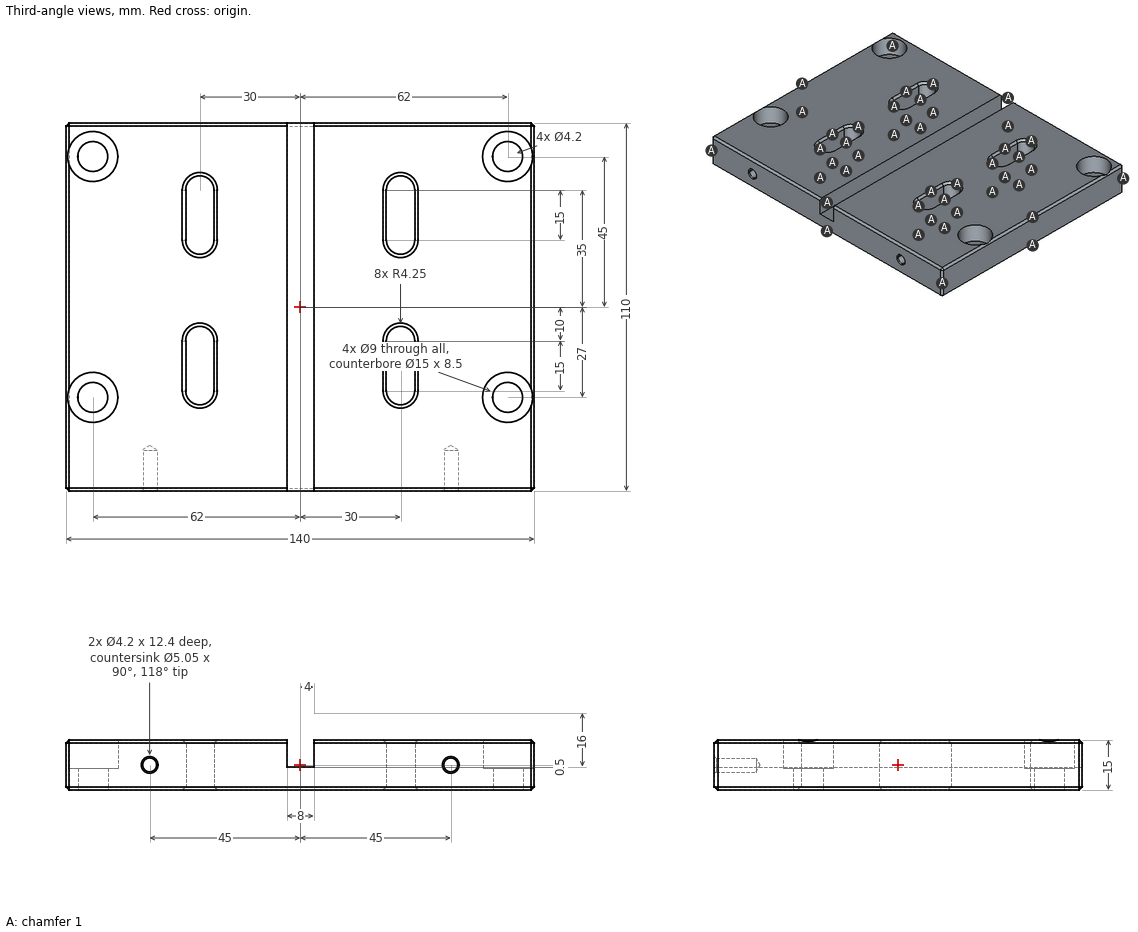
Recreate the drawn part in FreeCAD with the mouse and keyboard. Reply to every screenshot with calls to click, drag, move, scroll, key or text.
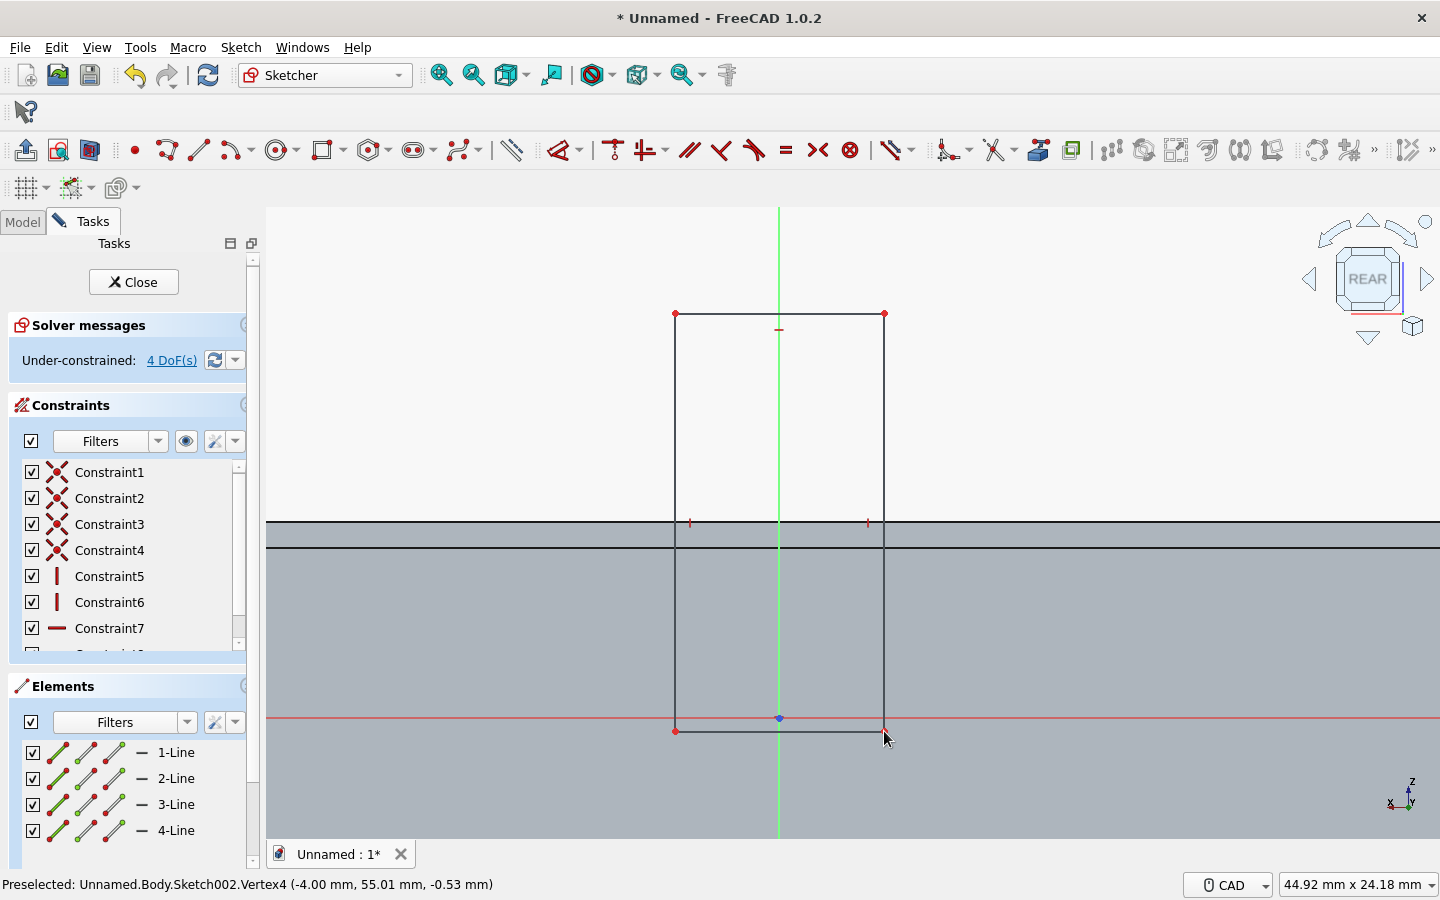
click(558, 150)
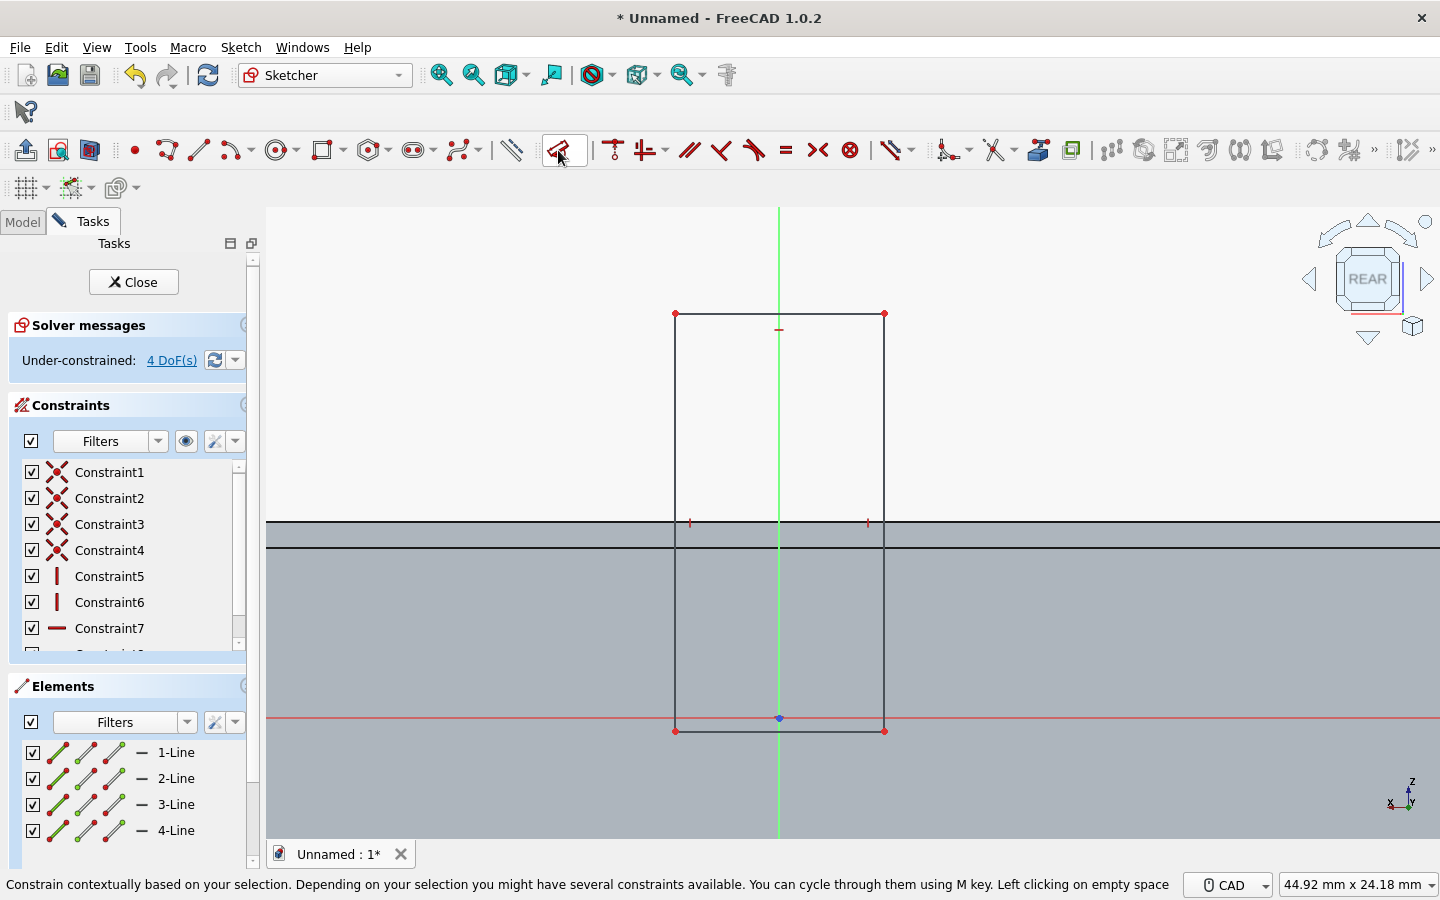
click(738, 732)
click(731, 766)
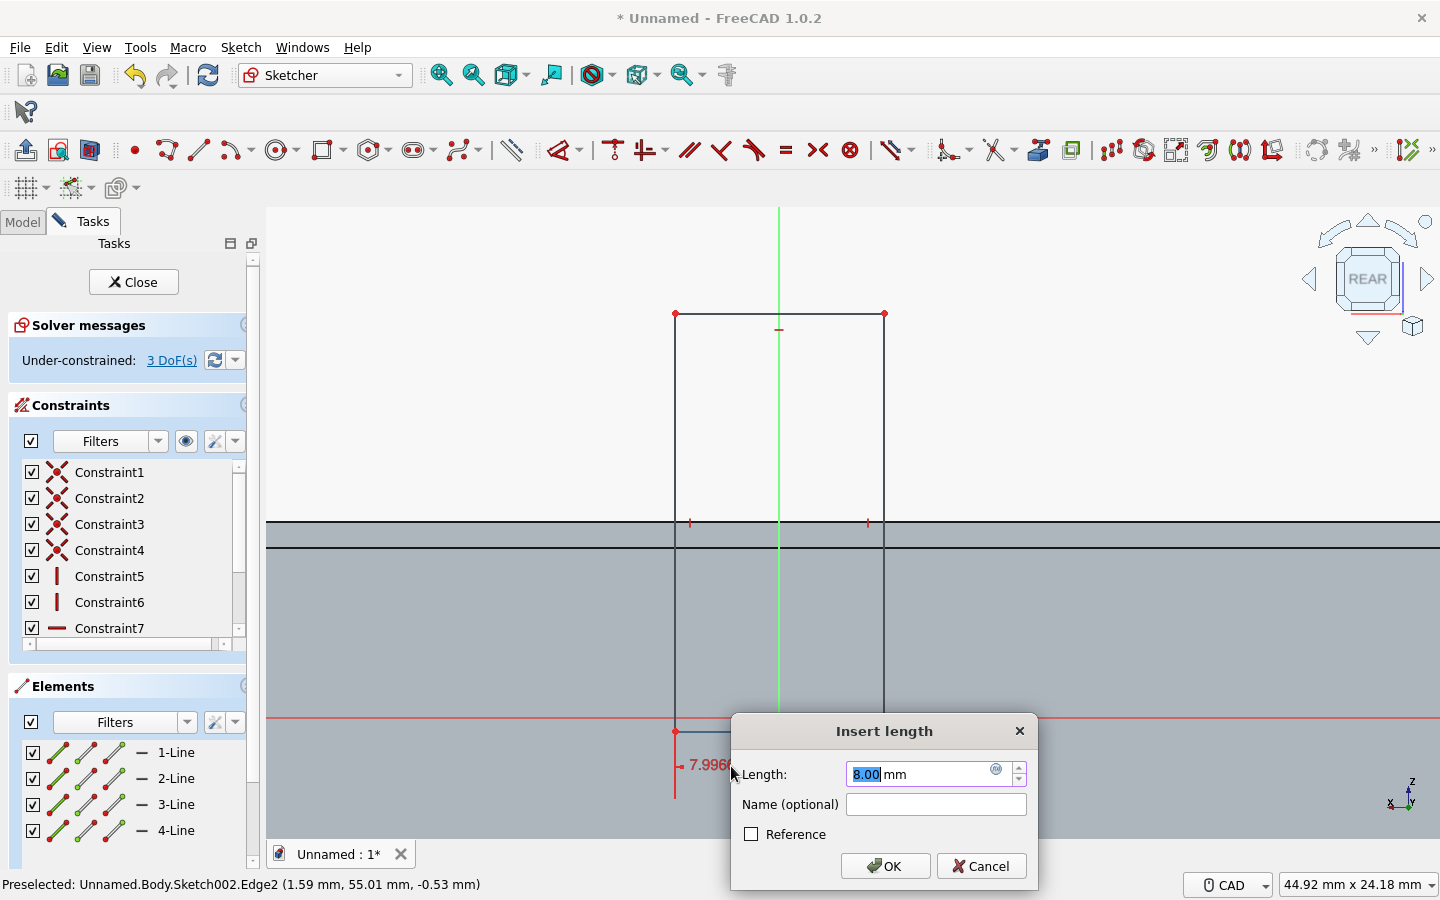
text(8)
key(Return)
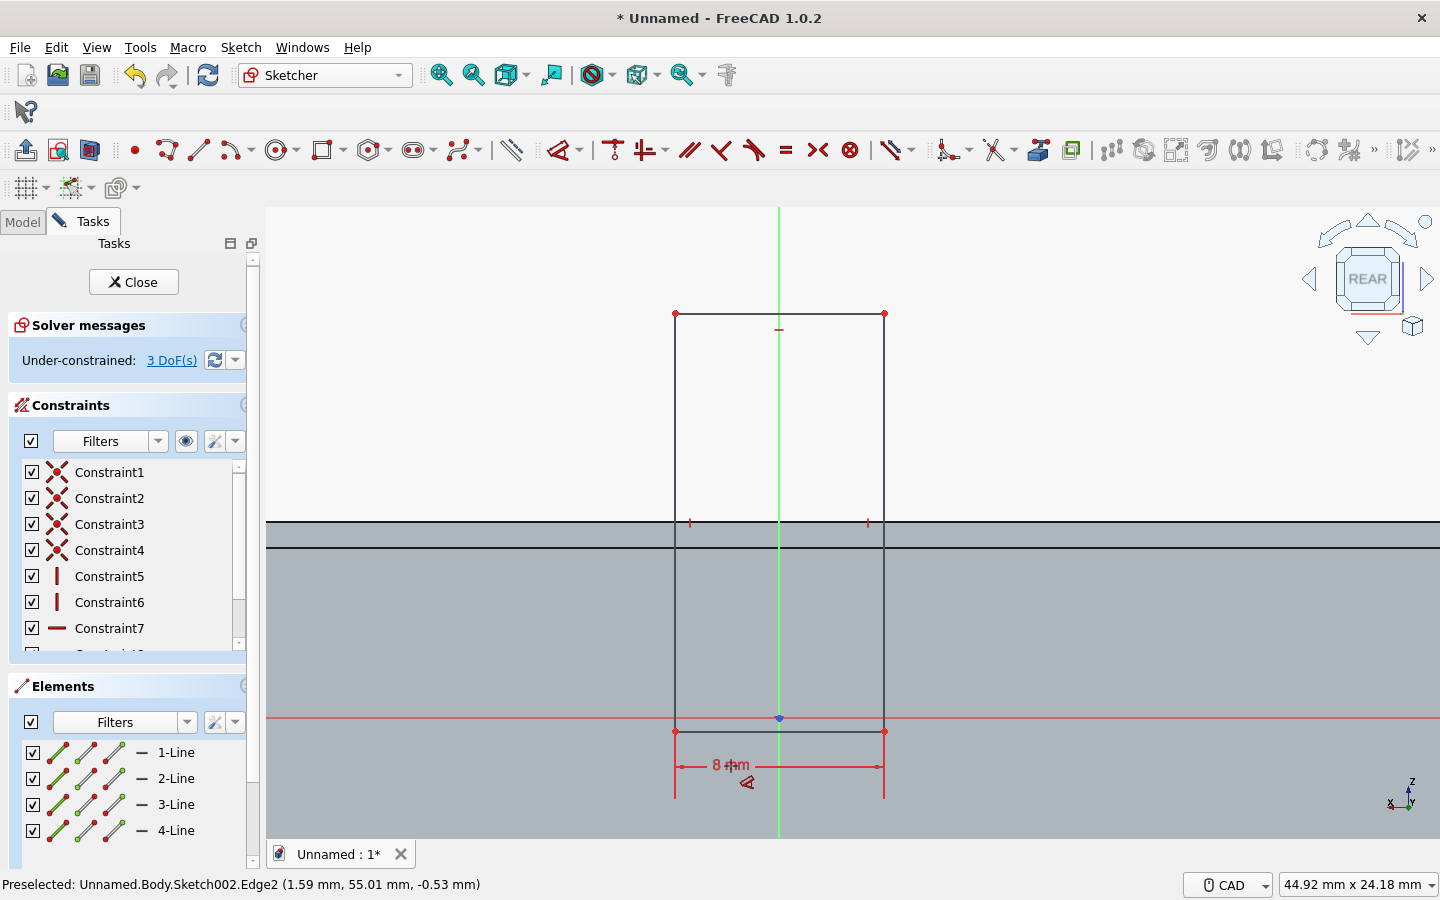
click(675, 439)
click(641, 523)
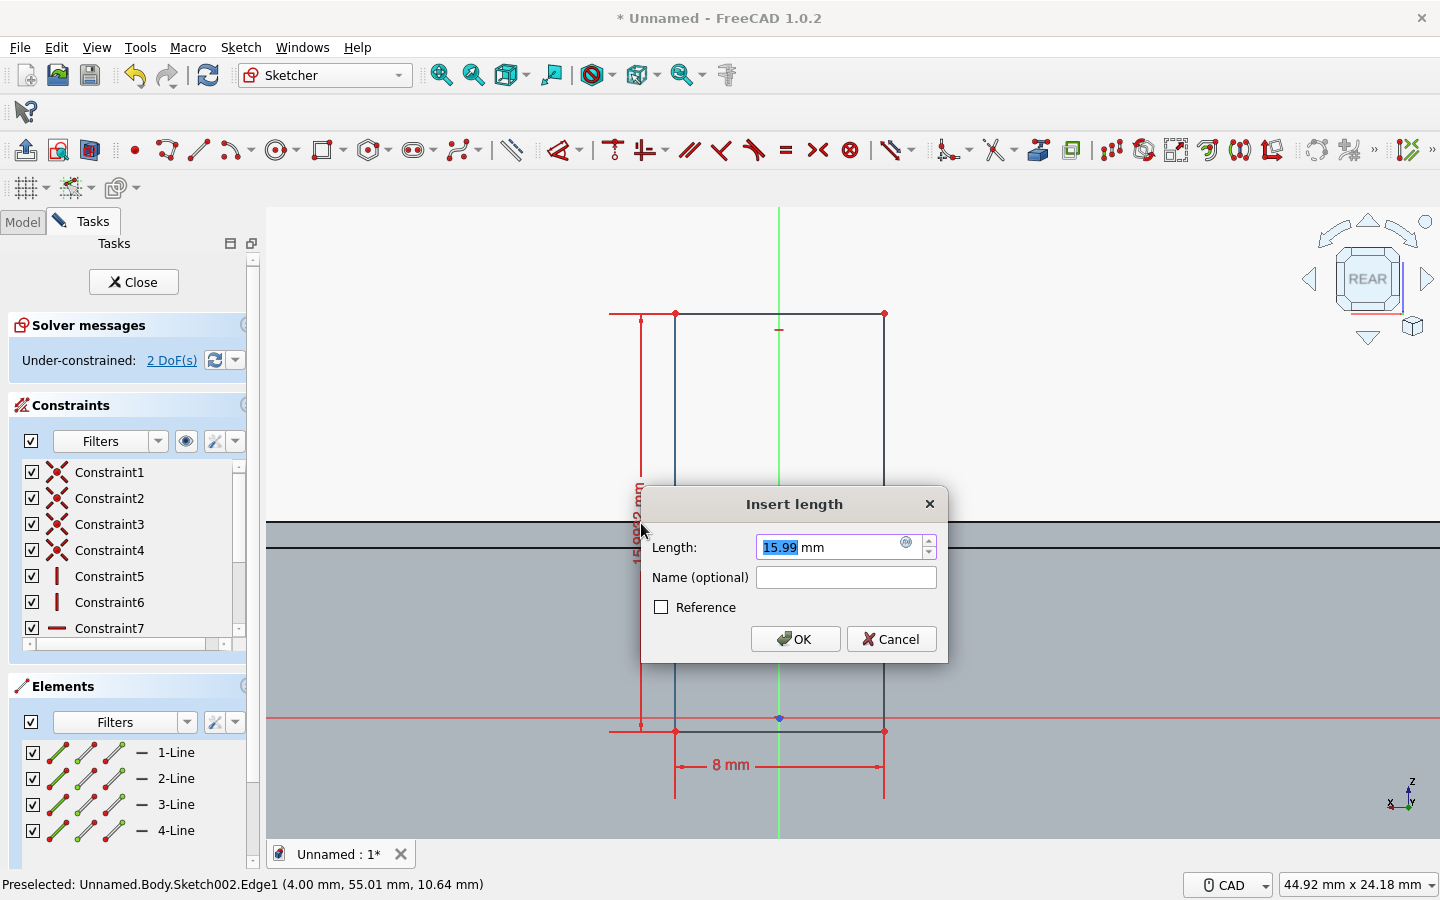
text(16)
key(Return)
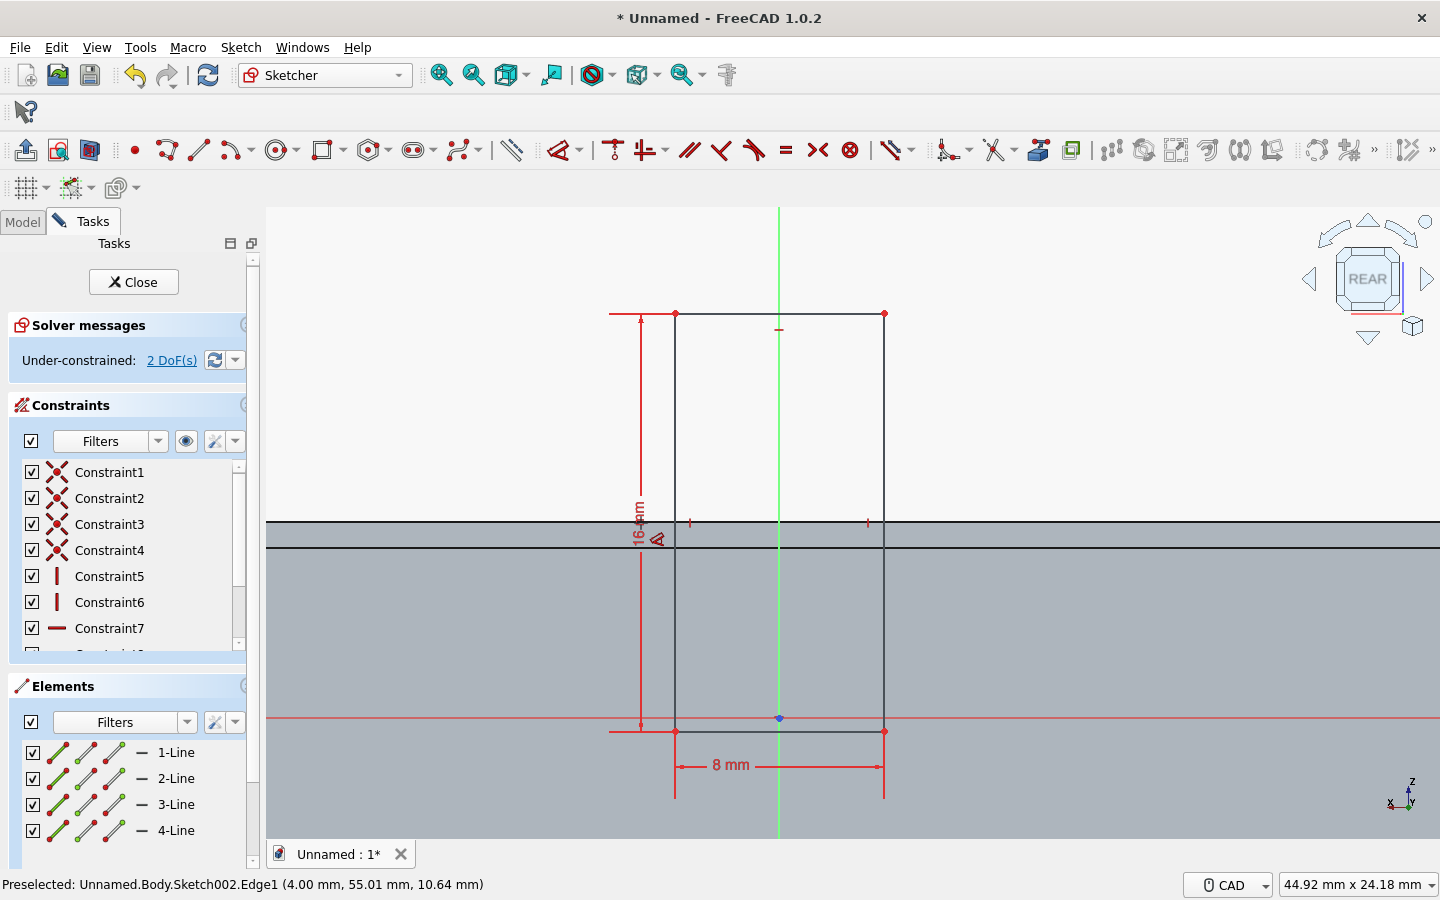
click(675, 314)
click(727, 280)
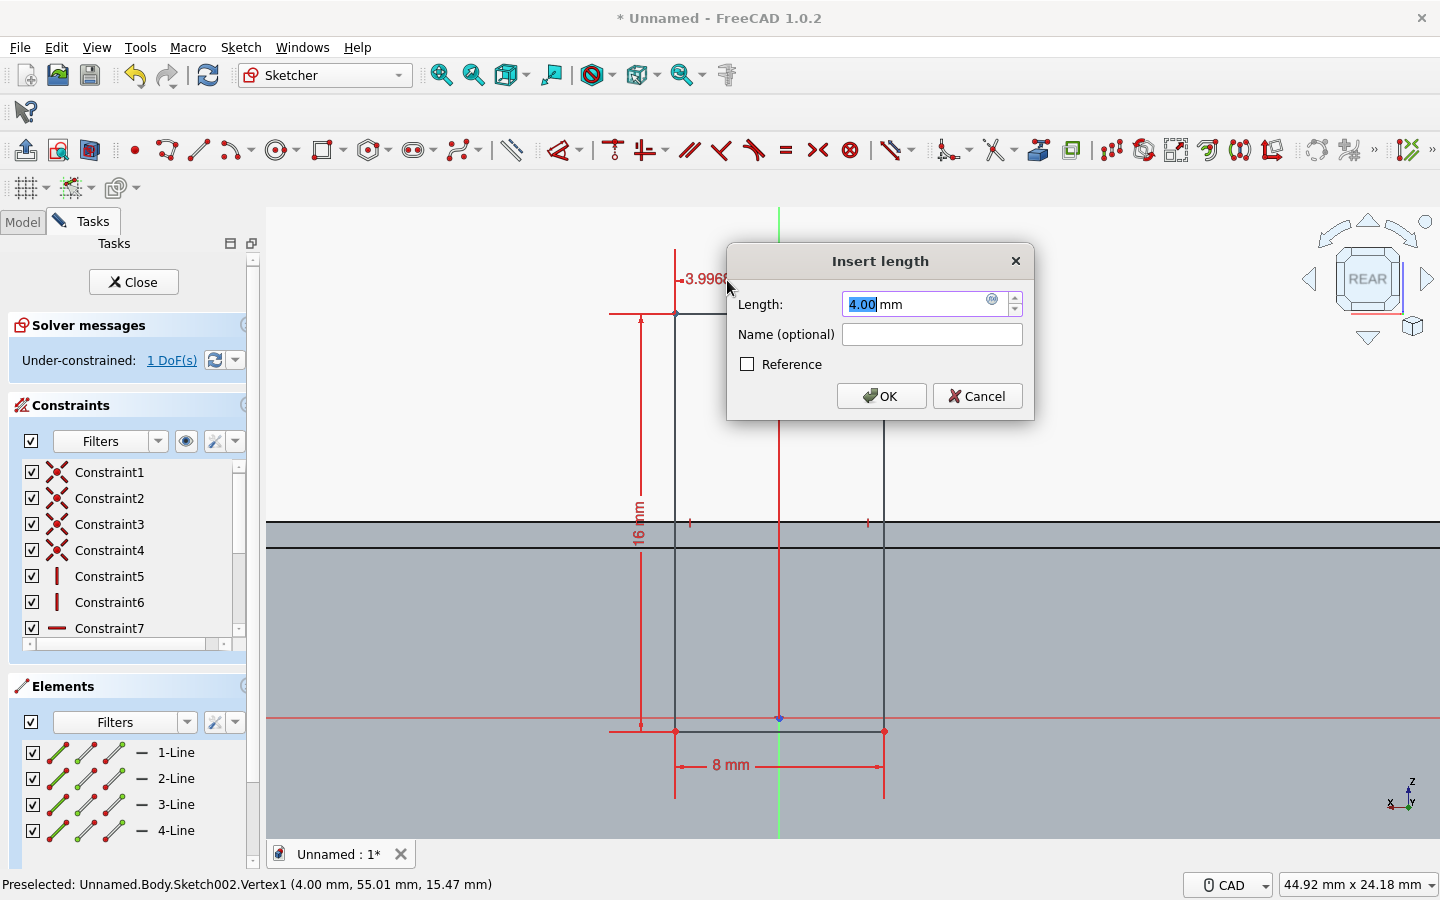
text(4)
key(Return)